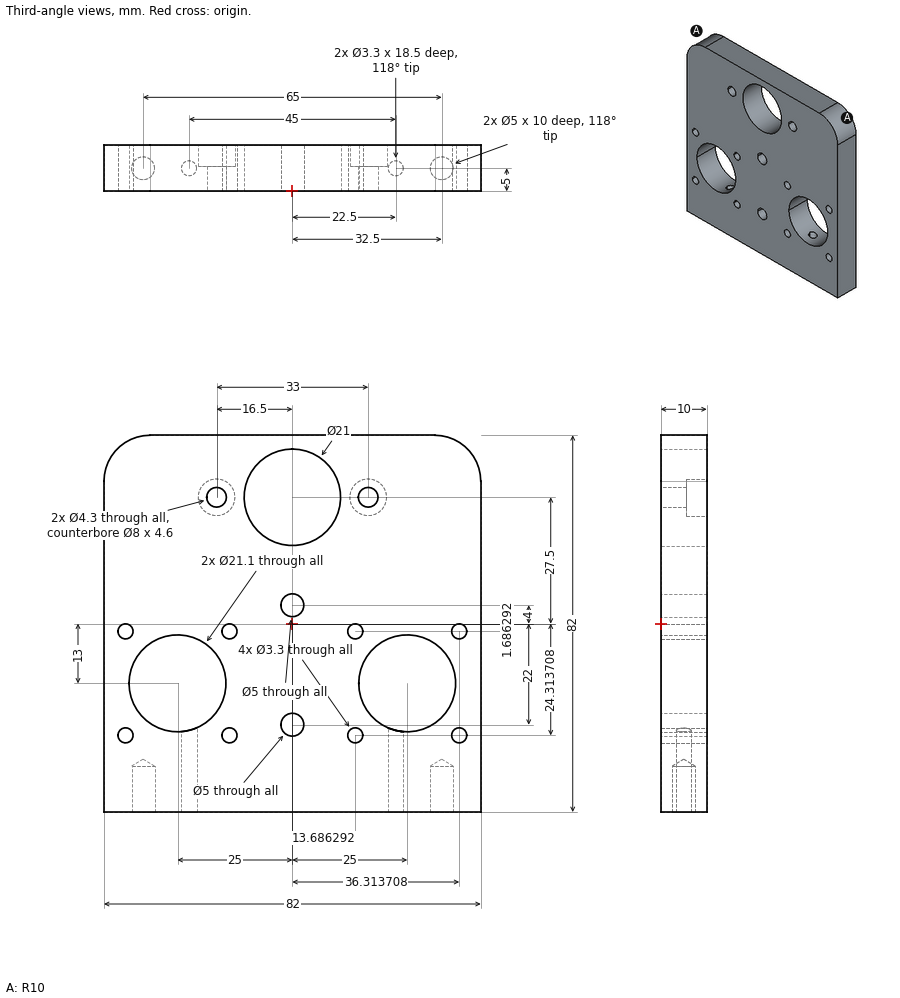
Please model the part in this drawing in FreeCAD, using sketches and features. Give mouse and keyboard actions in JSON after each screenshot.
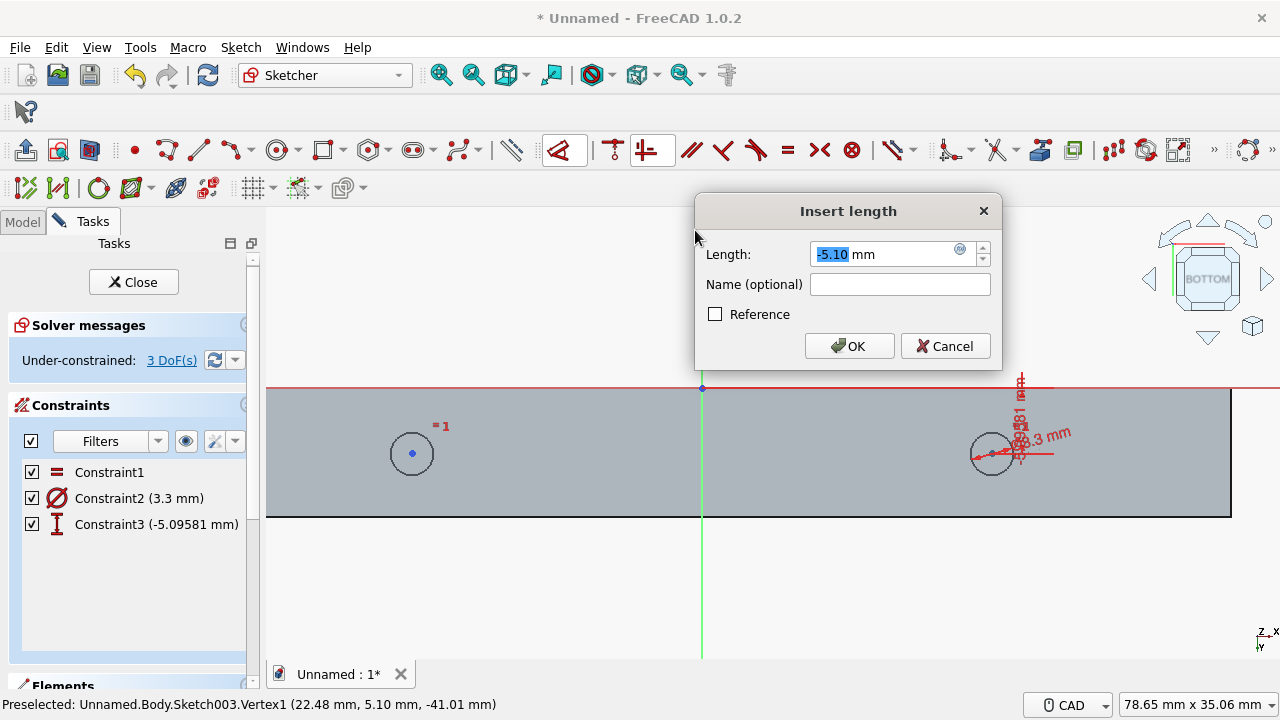
{"action": "type", "text": "-5"}
{"action": "key", "text": "Return"}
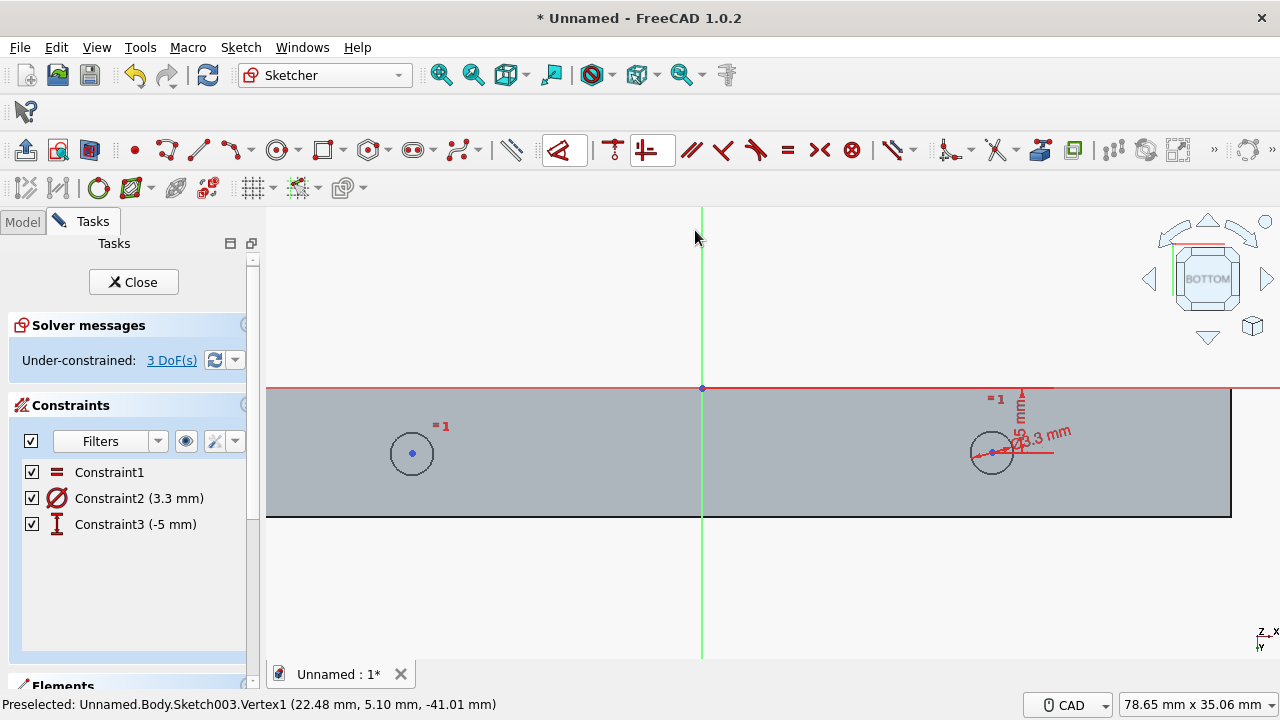
{"action": "left_click", "coordinate": [412, 454]}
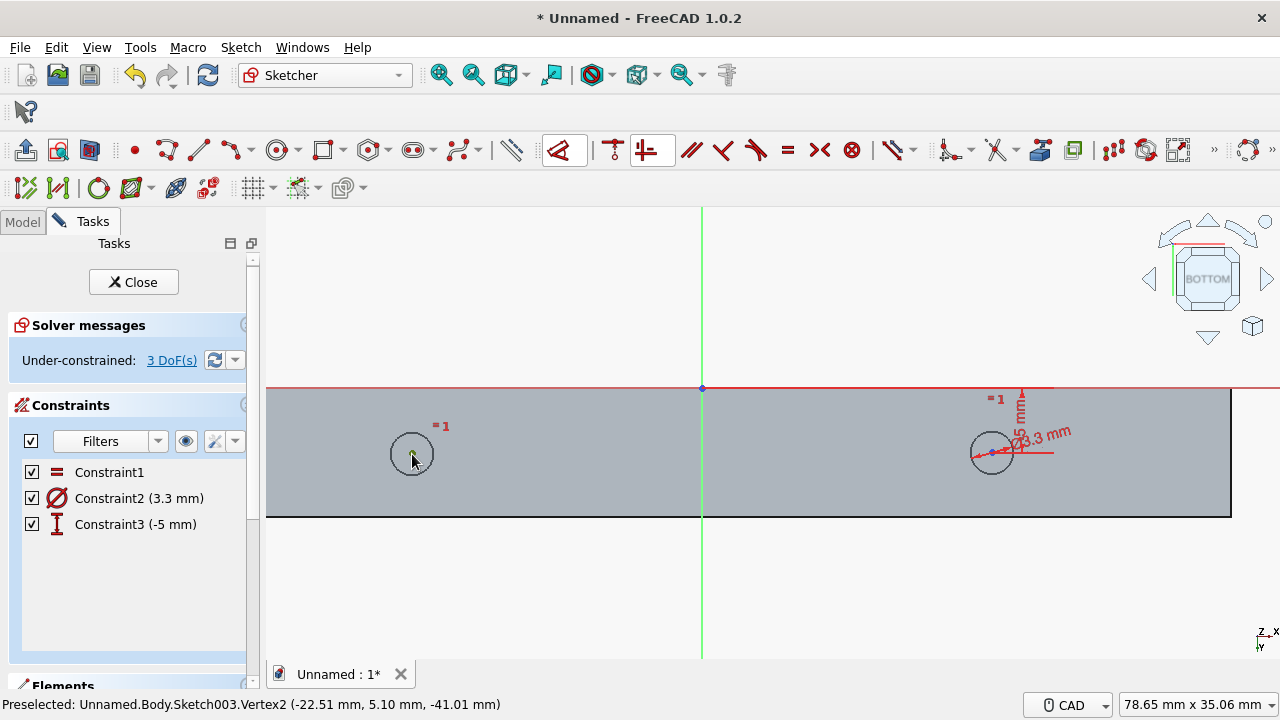
{"action": "left_click", "coordinate": [582, 150]}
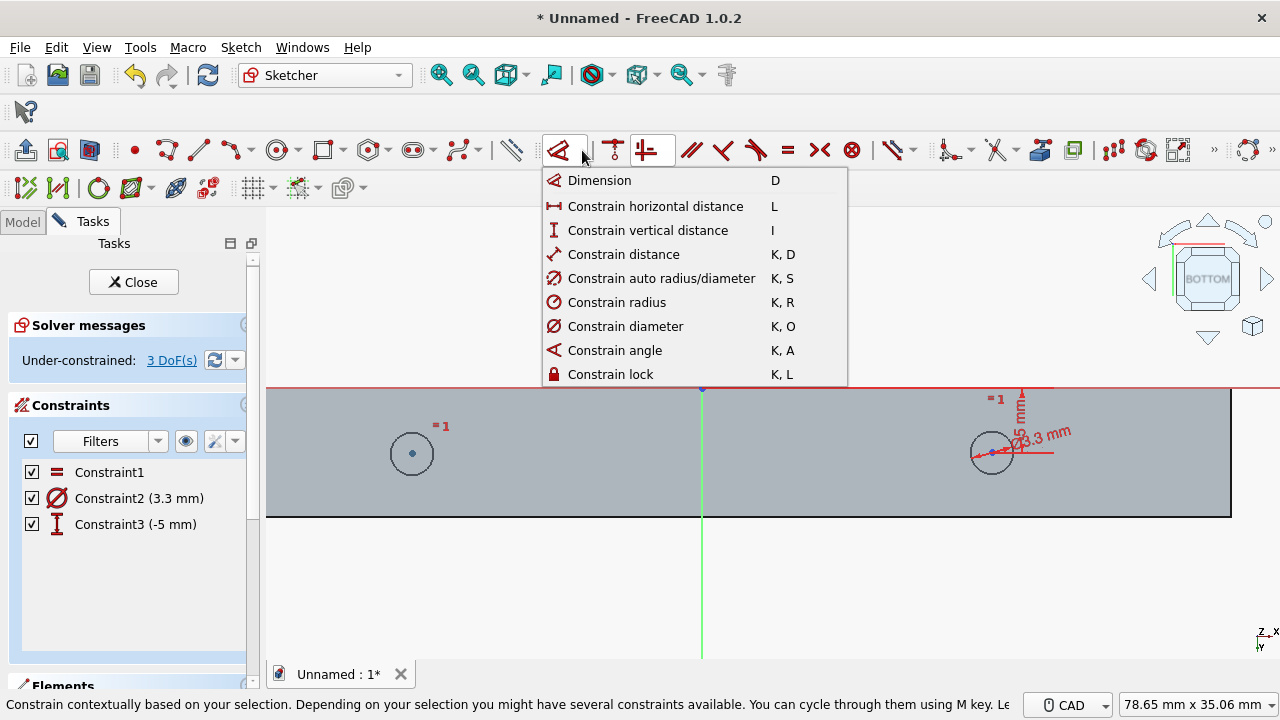
{"action": "left_click", "coordinate": [695, 230]}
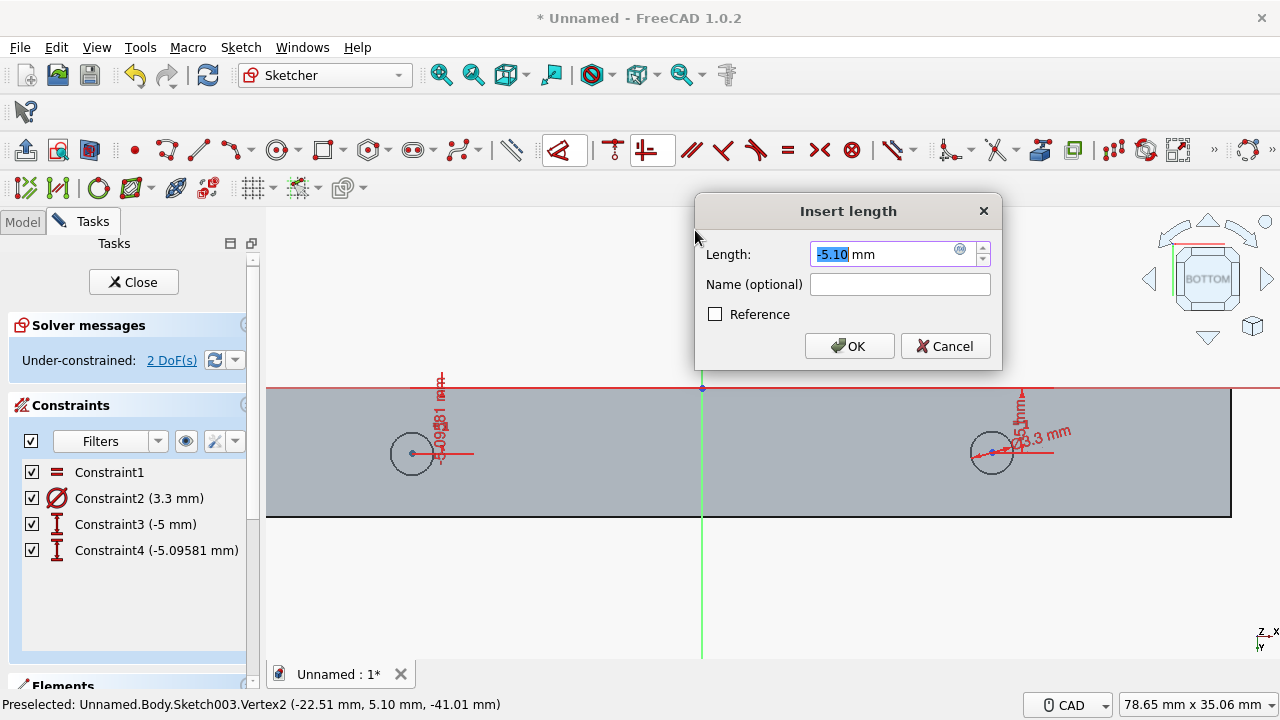
{"action": "type", "text": "-5"}
{"action": "key", "text": "Return"}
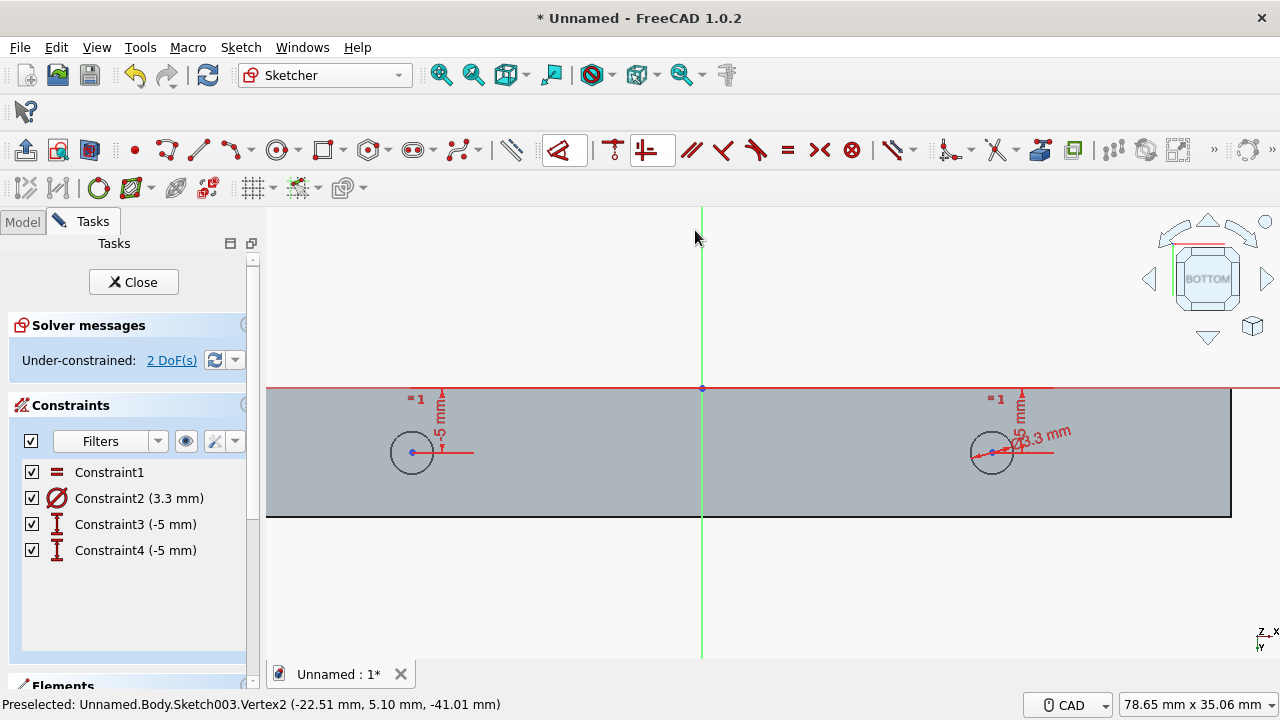
{"action": "left_click", "coordinate": [992, 453]}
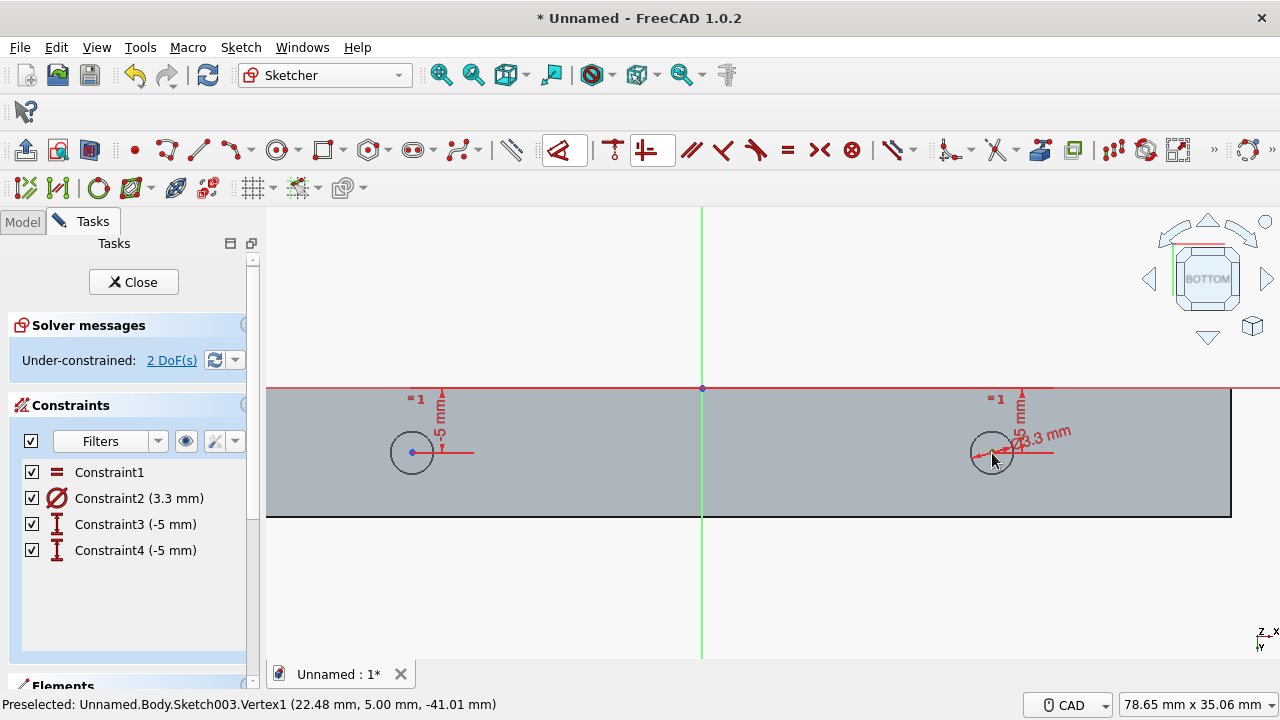
{"action": "left_click", "coordinate": [412, 453]}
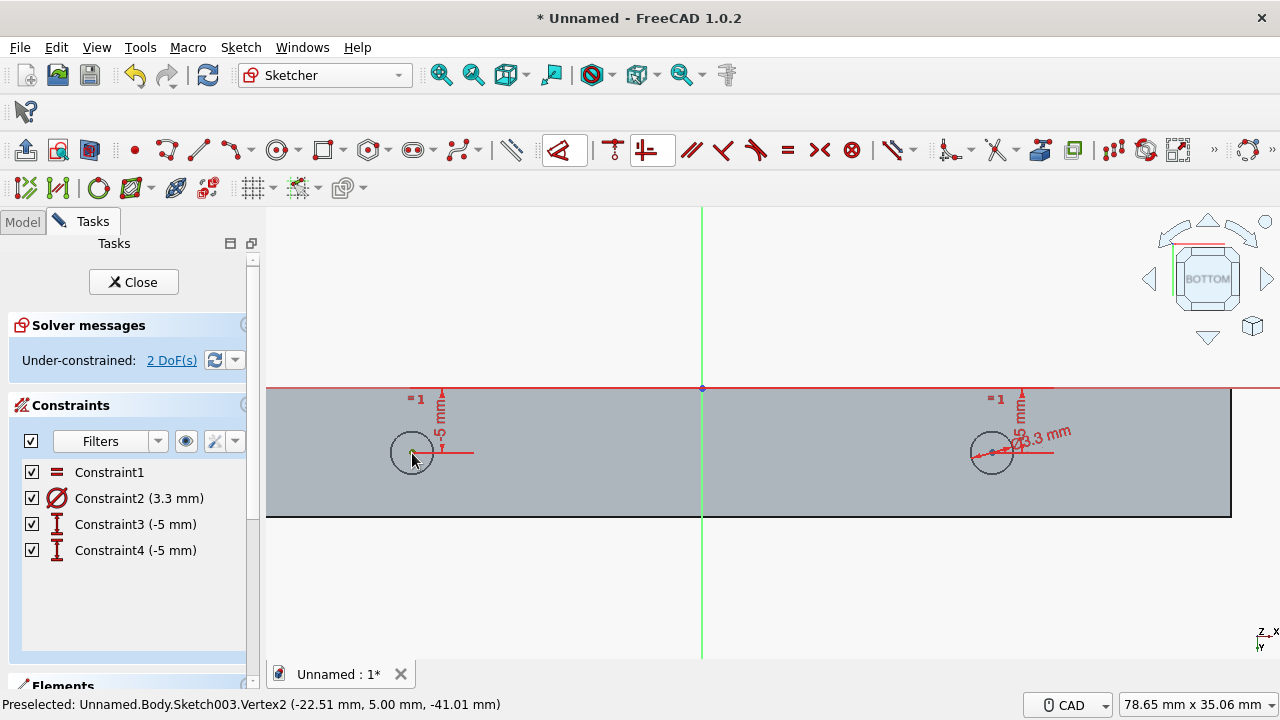
{"action": "key", "text": "l"}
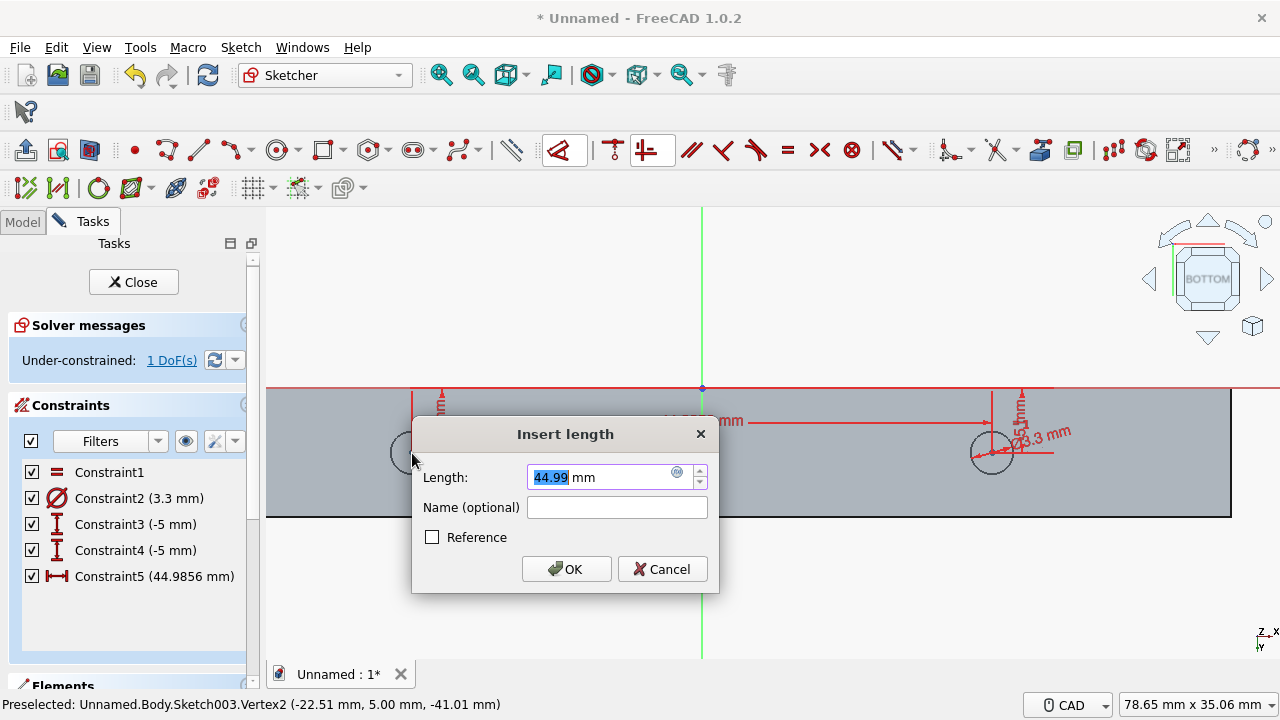
{"action": "type", "text": "45"}
{"action": "key", "text": "Return"}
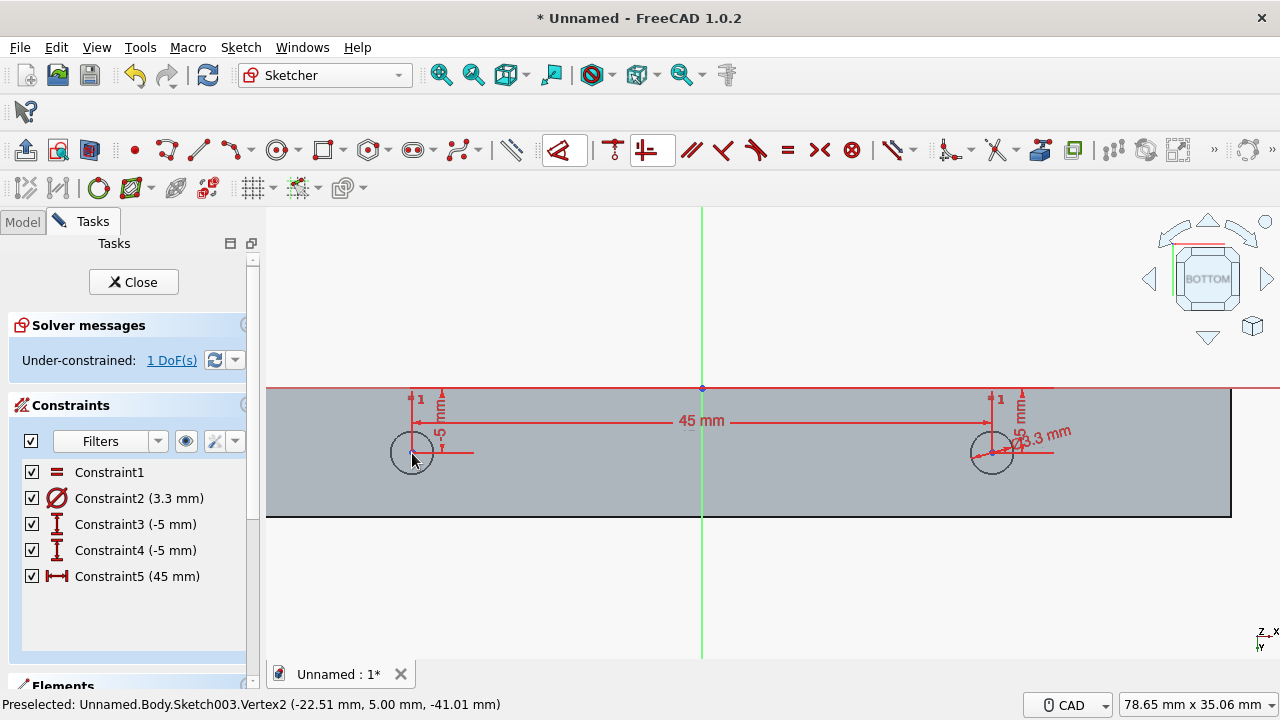
{"action": "left_click", "coordinate": [992, 453]}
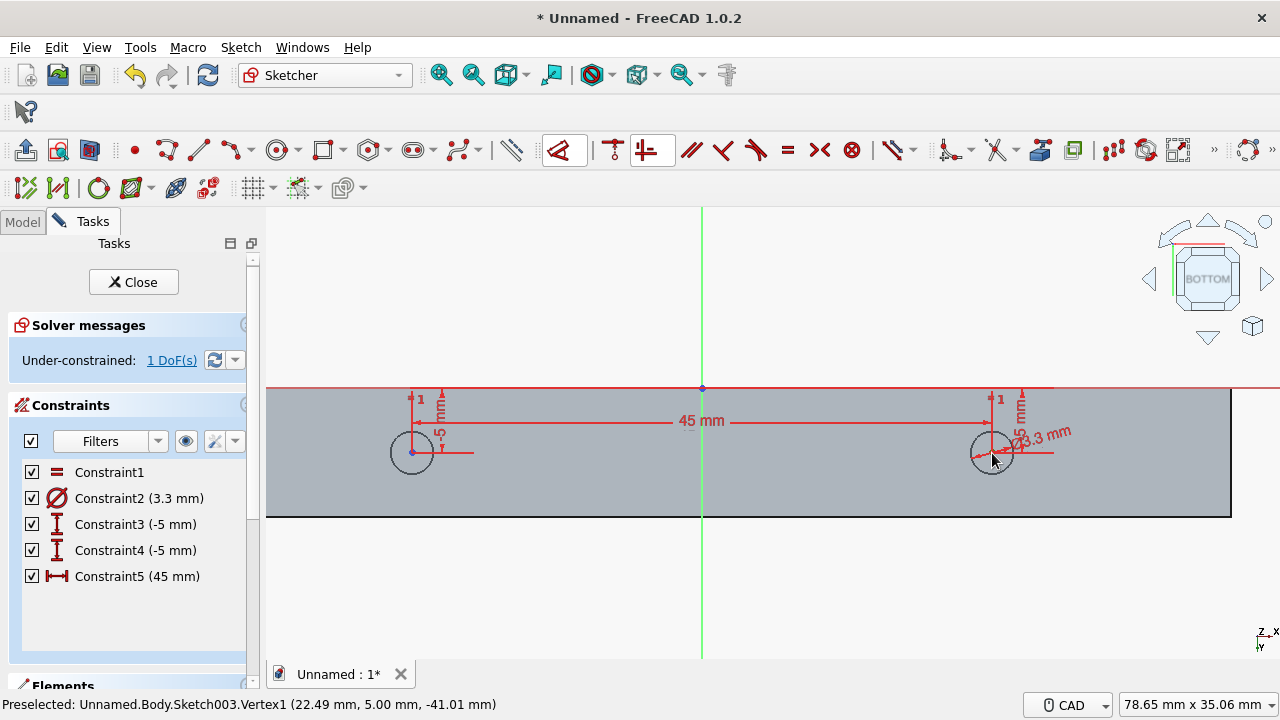
{"action": "left_click", "coordinate": [582, 150]}